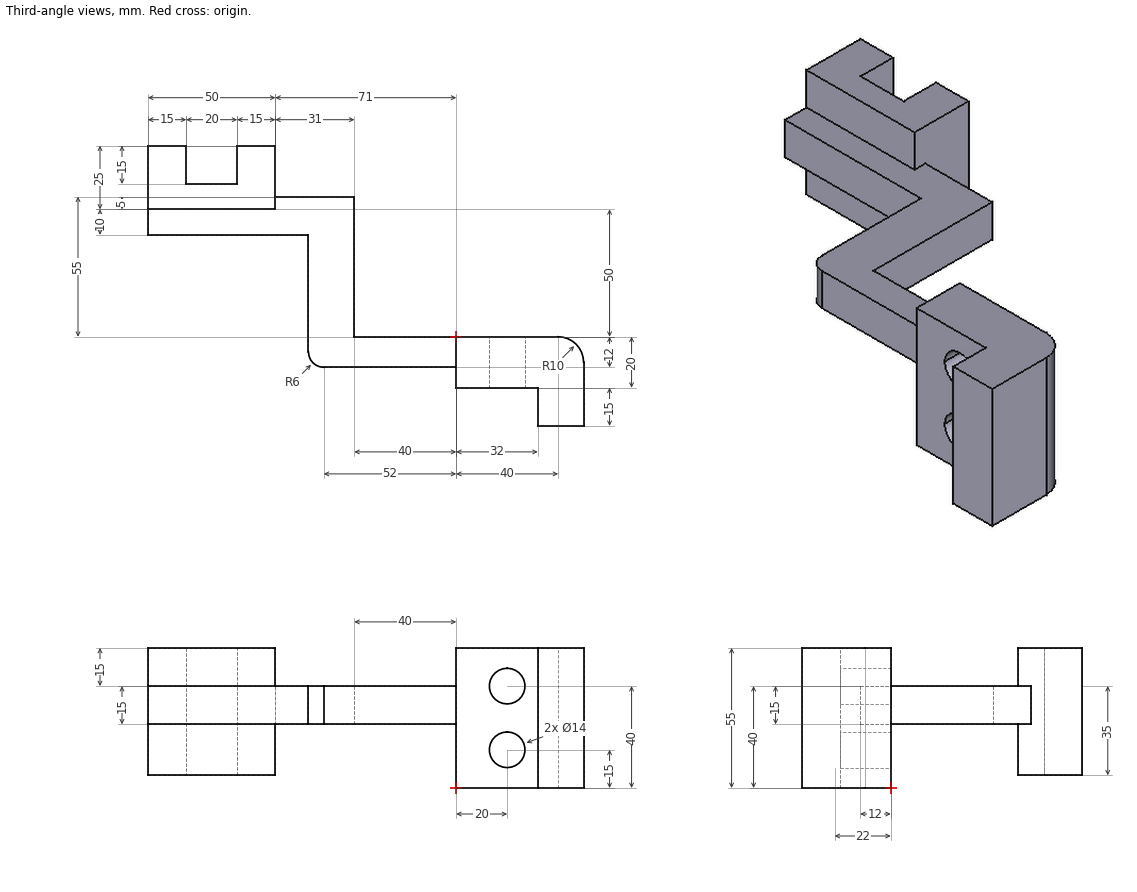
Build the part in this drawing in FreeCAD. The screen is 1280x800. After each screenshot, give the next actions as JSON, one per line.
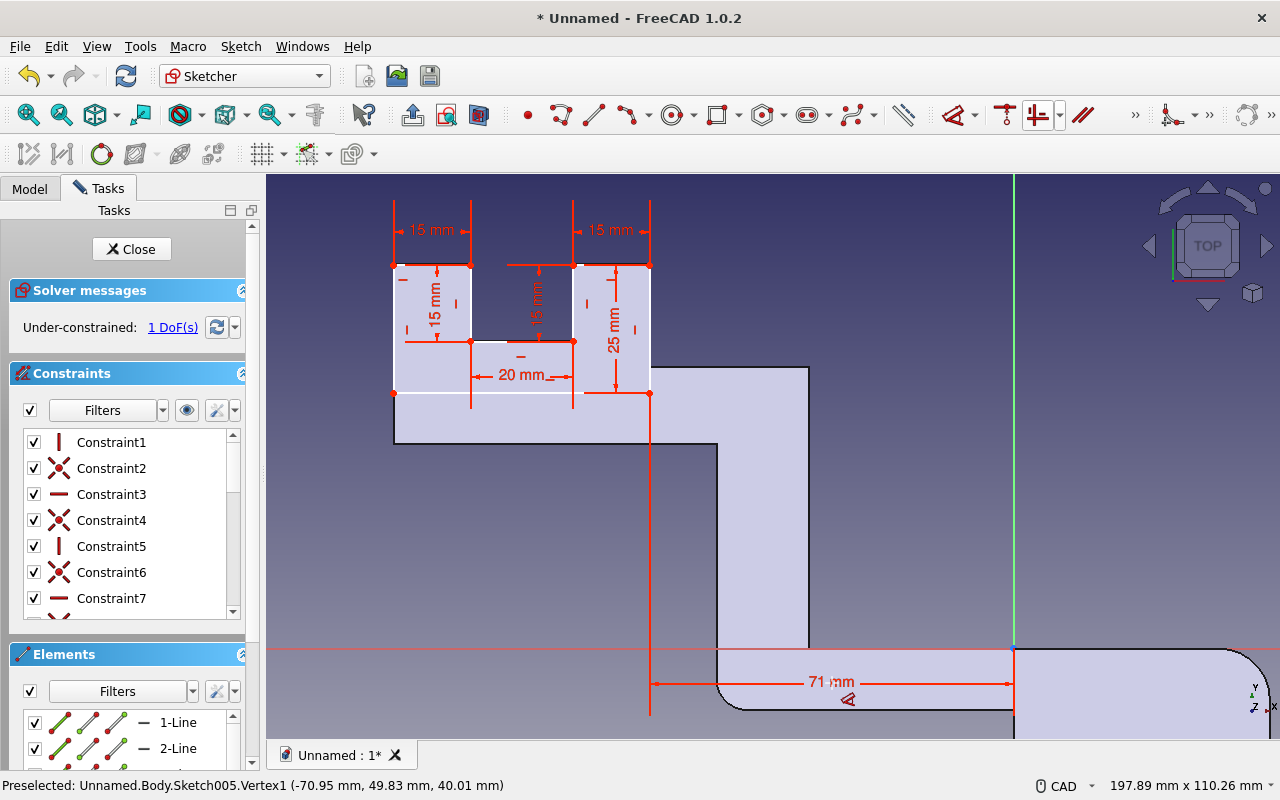
{"action": "left_click", "coordinate": [650, 393]}
{"action": "left_click", "coordinate": [1048, 521]}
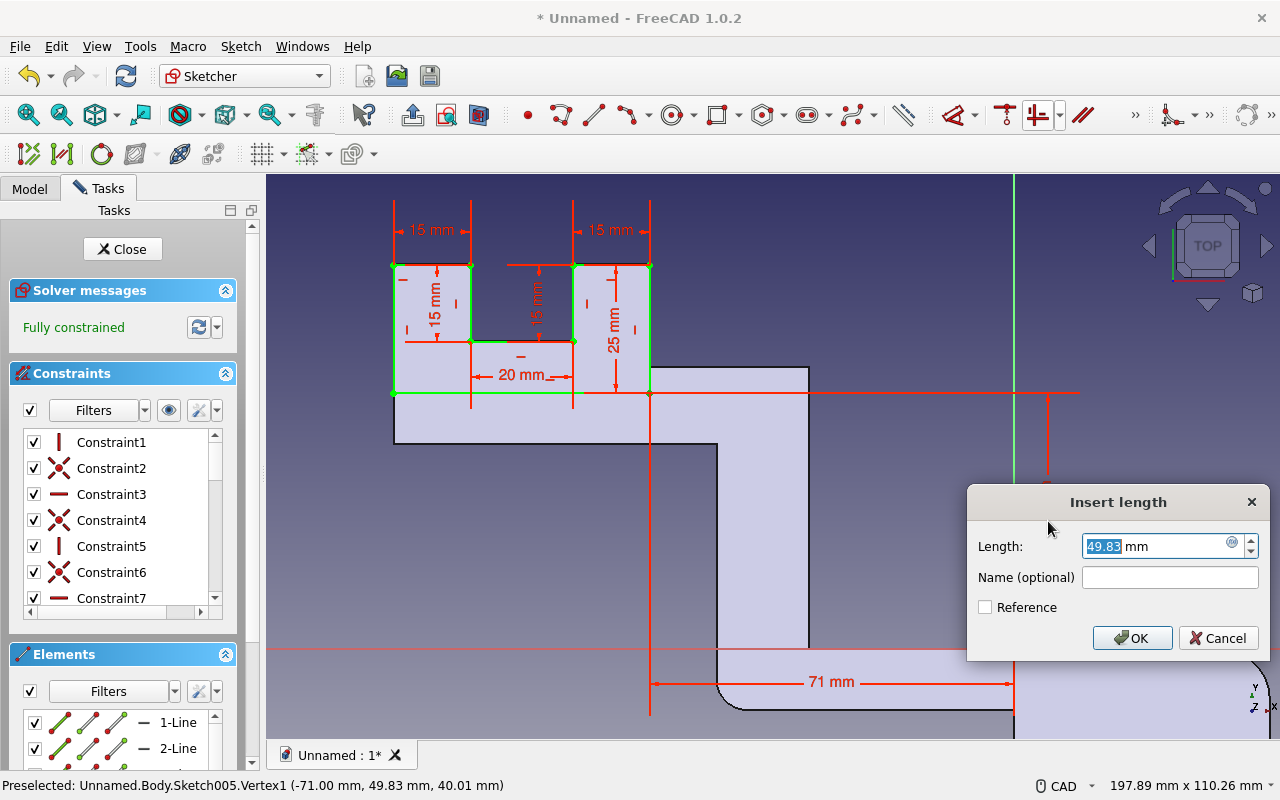
{"action": "type", "text": "50"}
{"action": "key", "text": "Return"}
{"action": "key", "text": "Escape"}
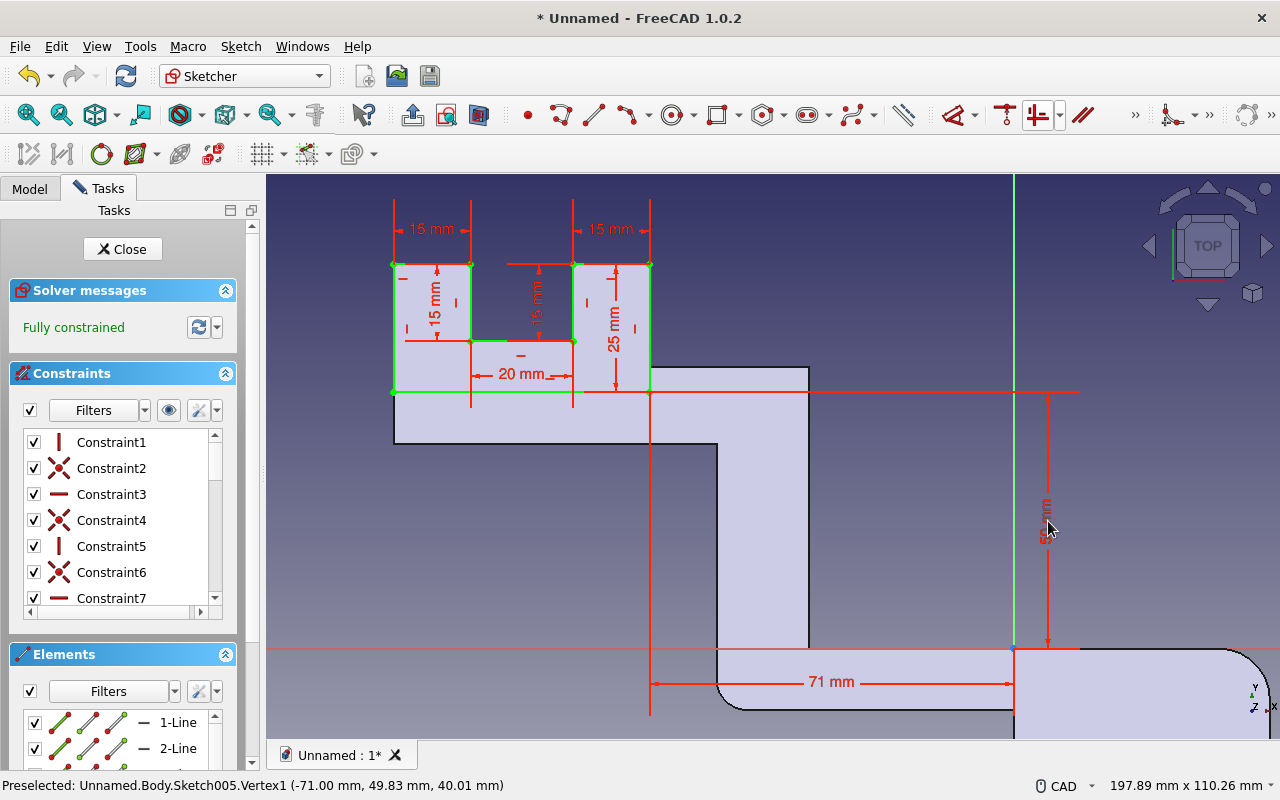
{"action": "left_click", "coordinate": [123, 249]}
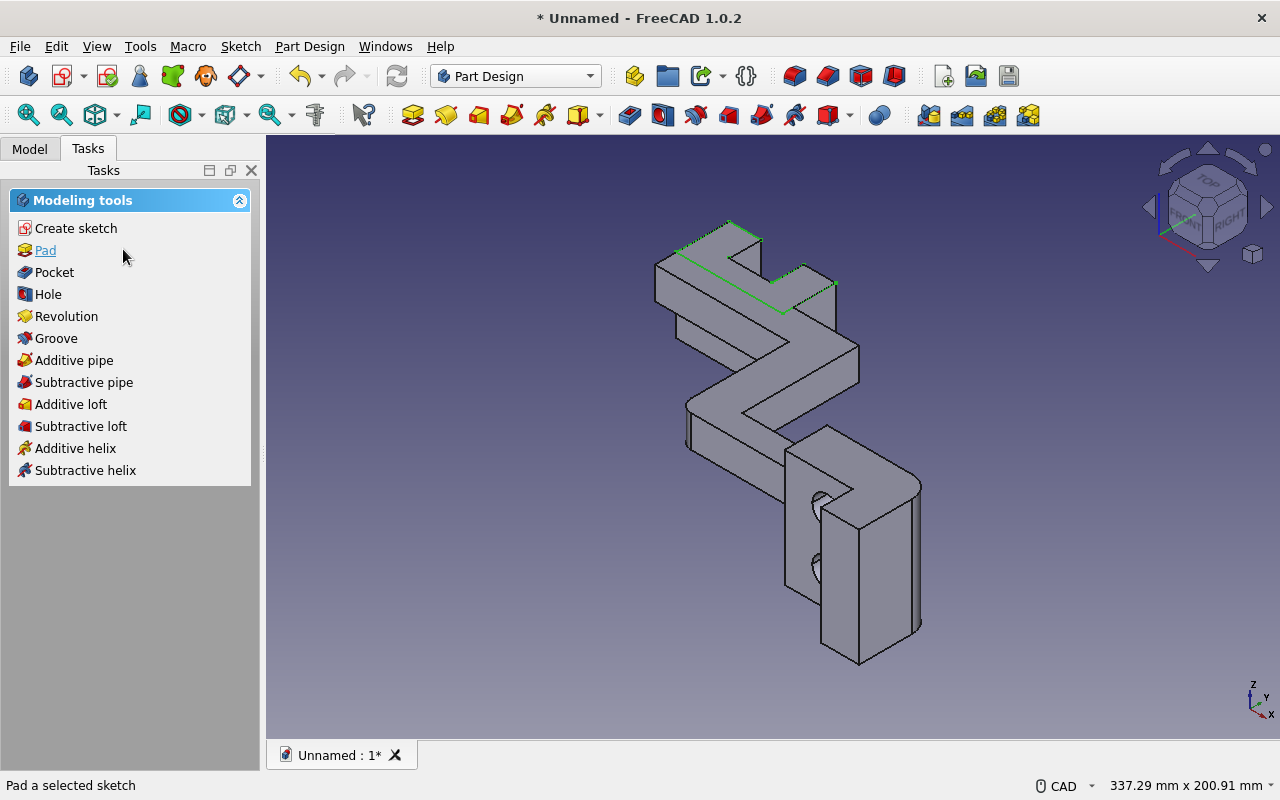
{"action": "left_click", "coordinate": [413, 116]}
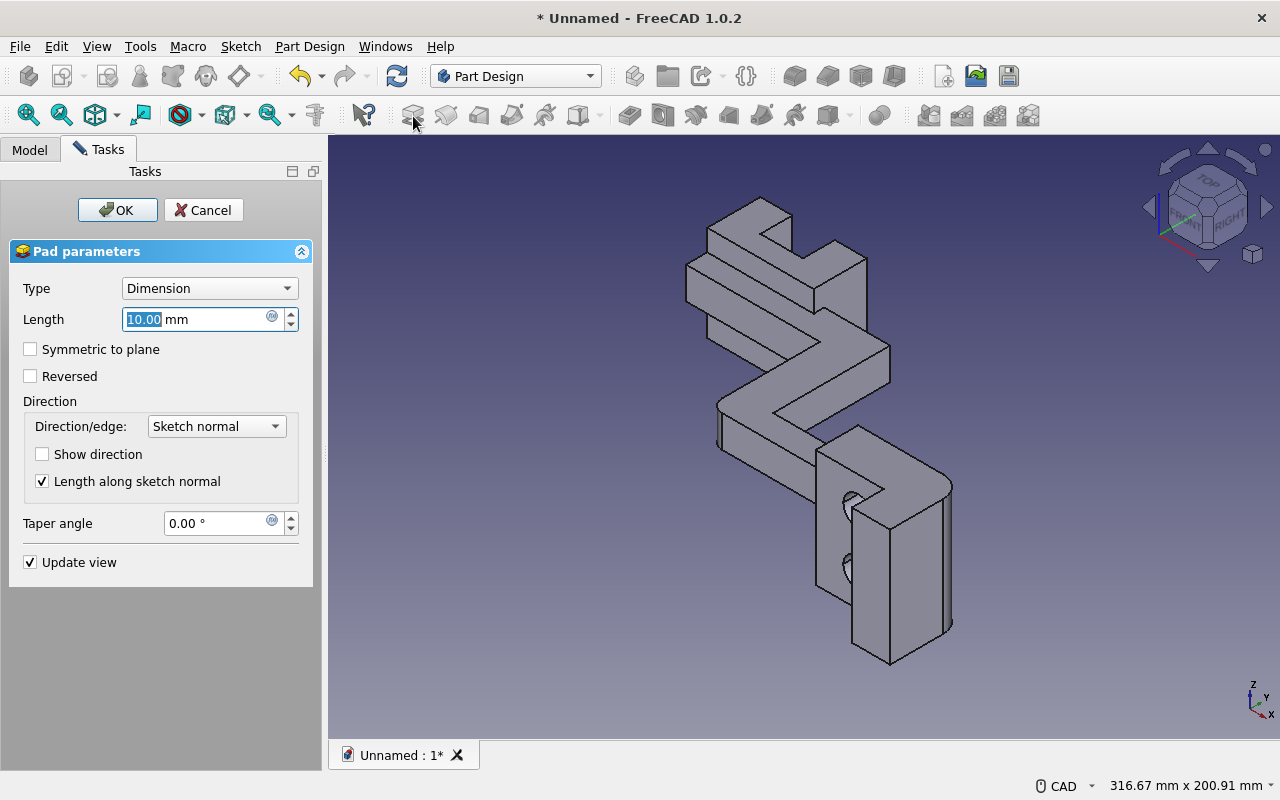
{"action": "type", "text": "15"}
{"action": "key", "text": "Tab"}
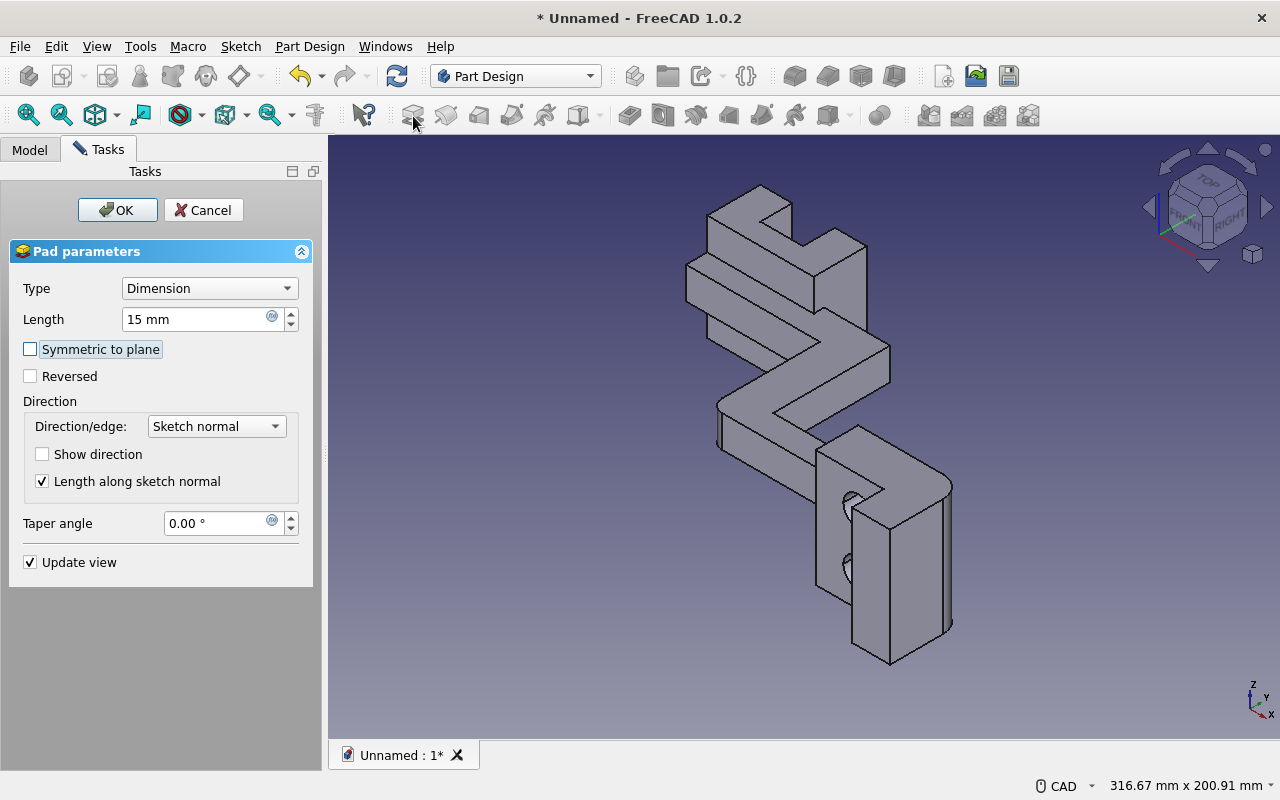
{"action": "left_click", "coordinate": [118, 210]}